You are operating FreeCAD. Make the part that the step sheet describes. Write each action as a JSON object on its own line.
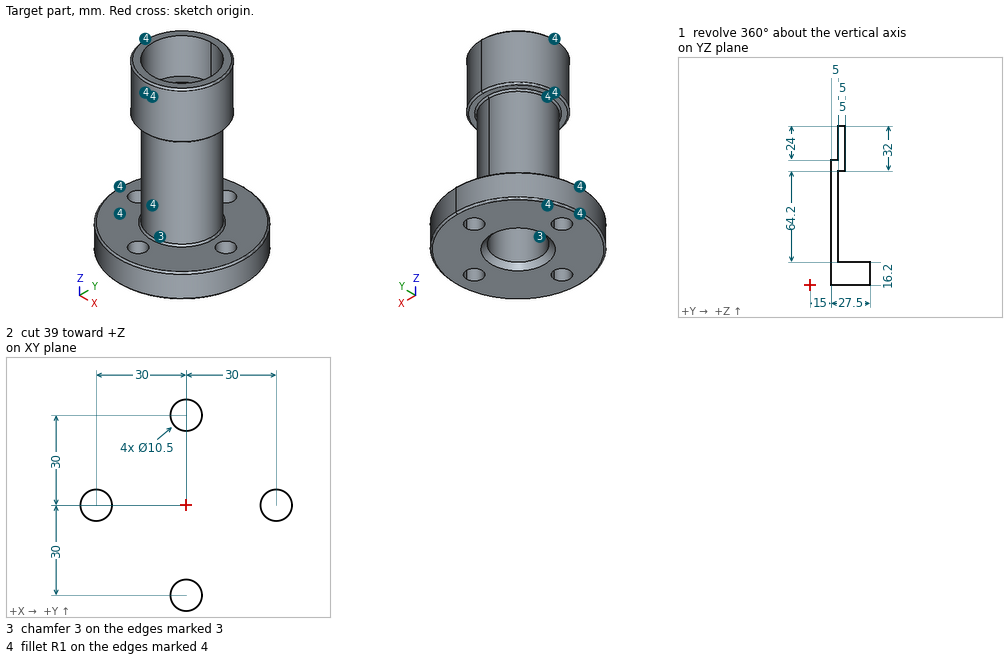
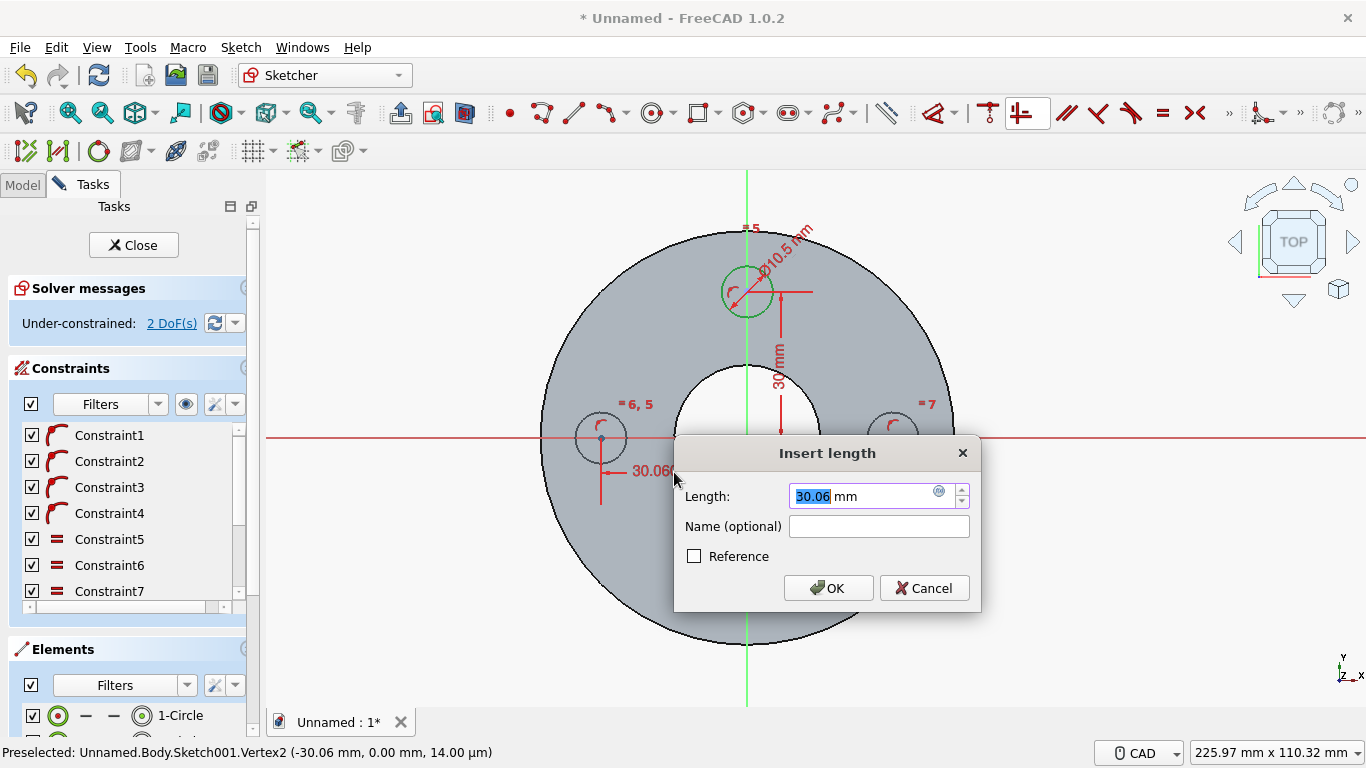
{"action": "type", "text": "30"}
{"action": "key", "text": "Return"}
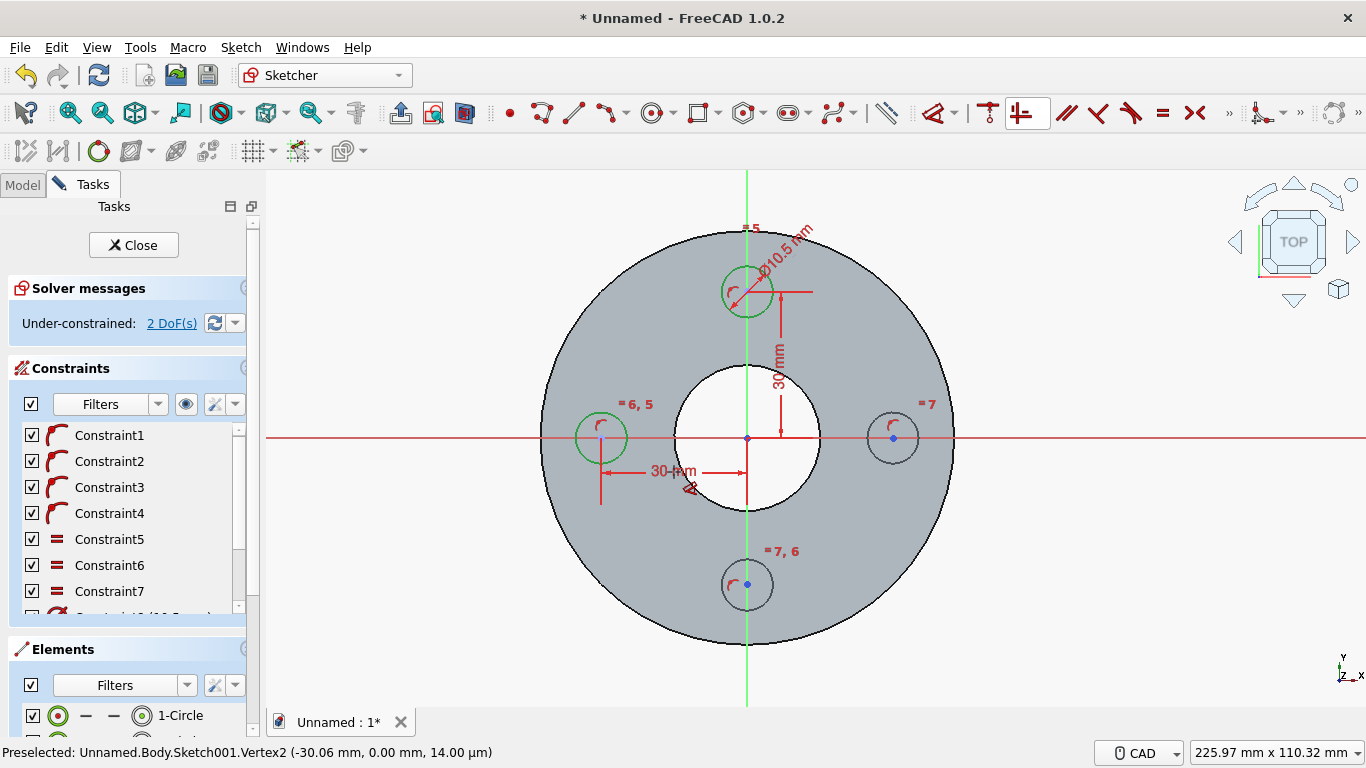
{"action": "left_click", "coordinate": [747, 585]}
{"action": "left_click", "coordinate": [781, 512]}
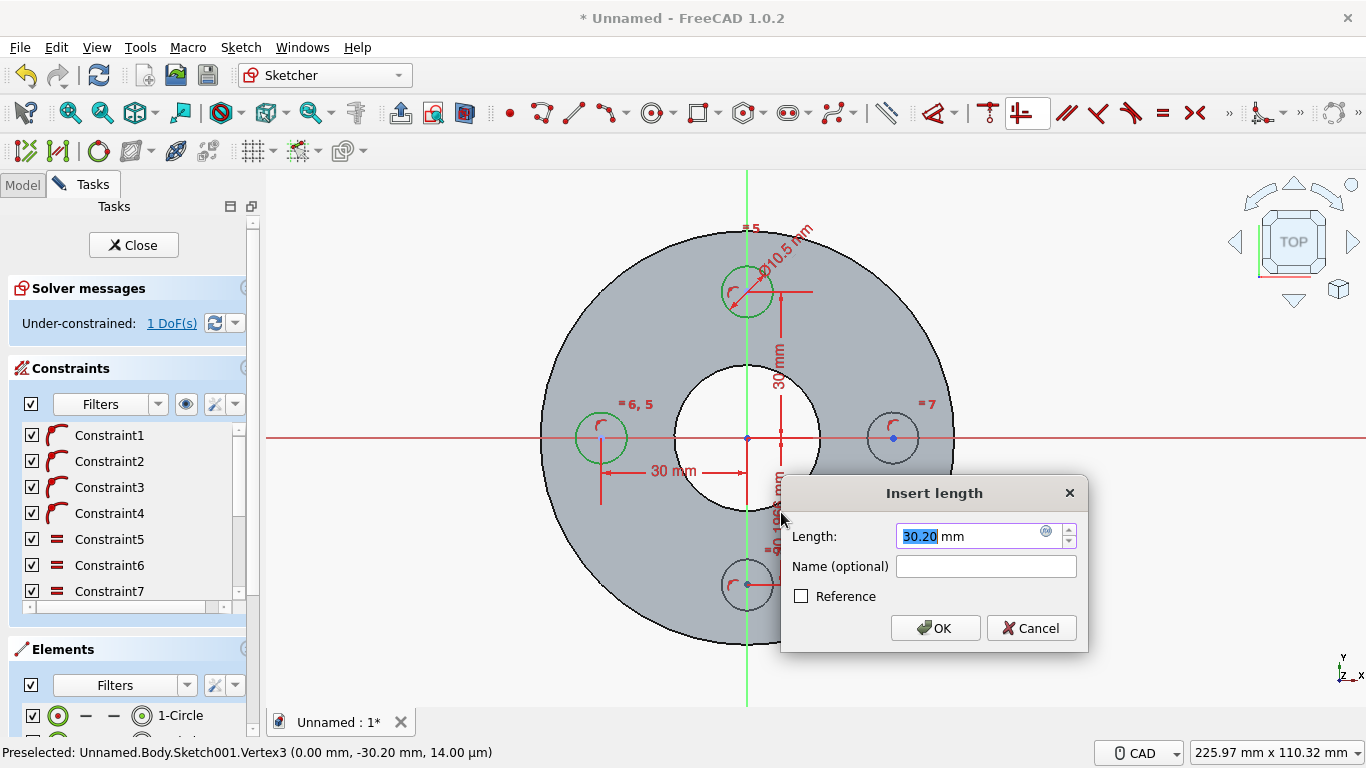
{"action": "type", "text": "30"}
{"action": "key", "text": "Return"}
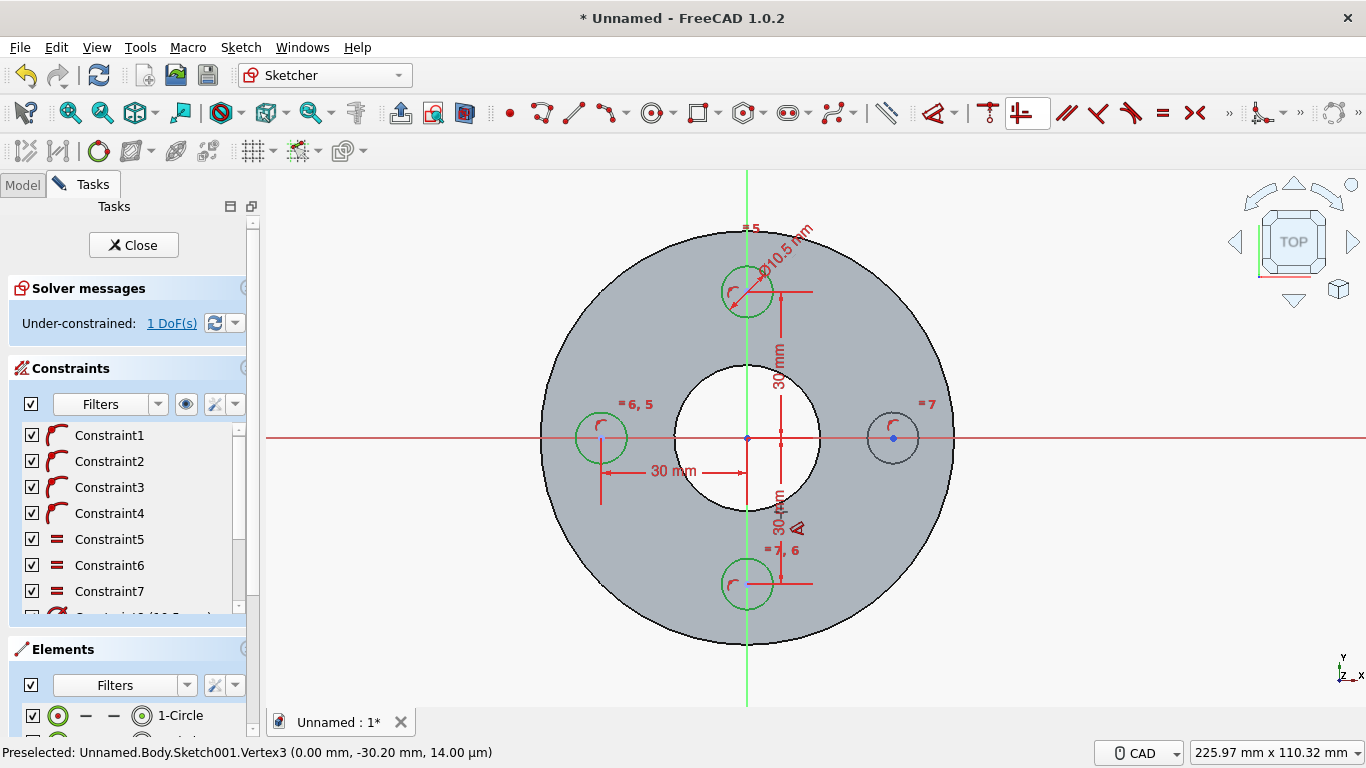
{"action": "left_click", "coordinate": [893, 438]}
{"action": "left_click", "coordinate": [820, 472]}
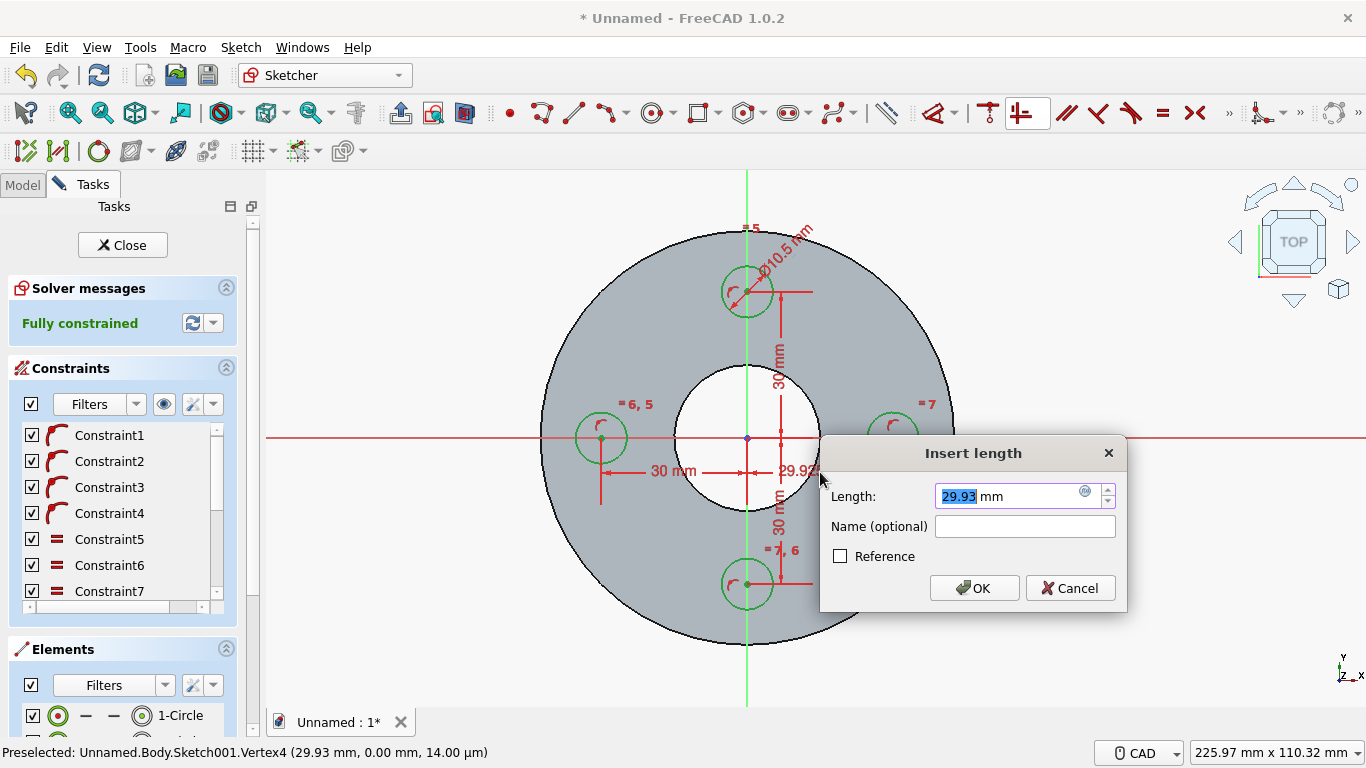
{"action": "type", "text": "30"}
{"action": "key", "text": "Return"}
{"action": "key", "text": "Escape"}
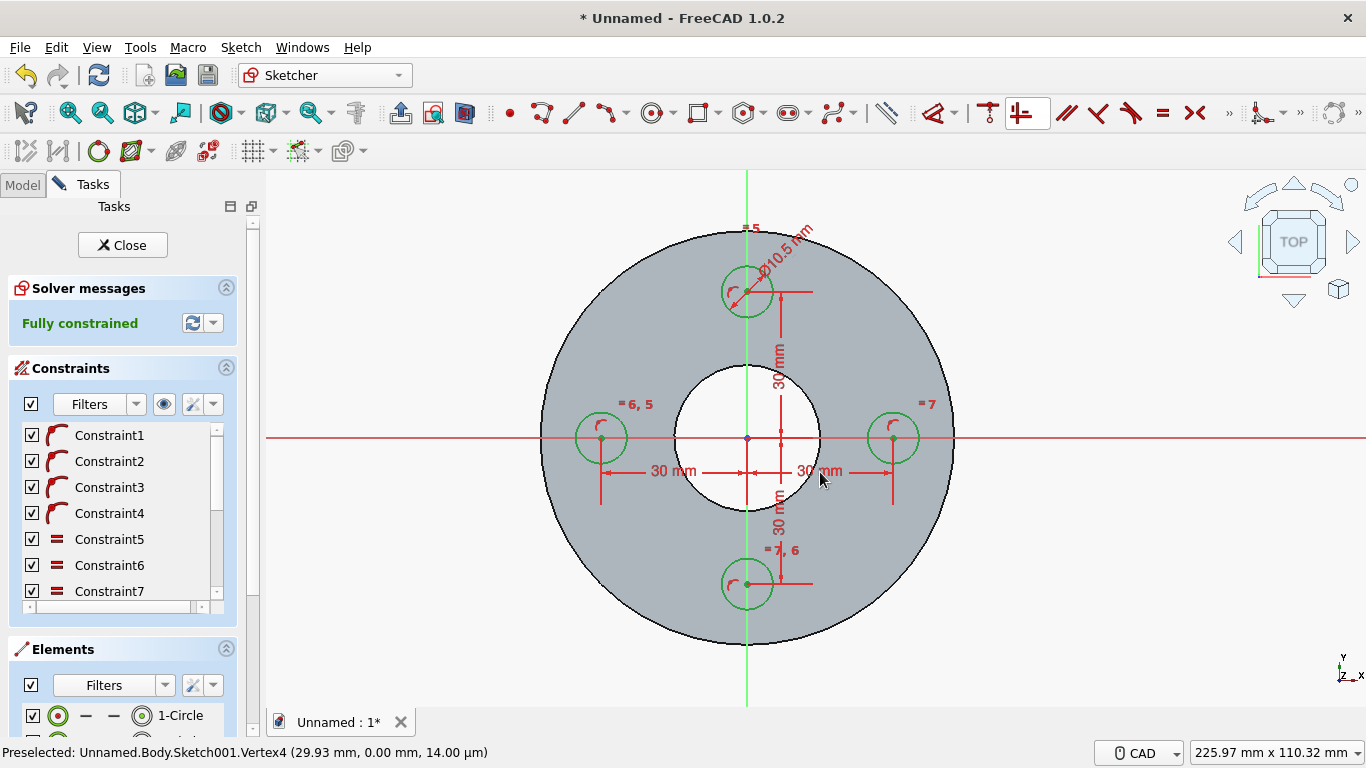
{"action": "left_click", "coordinate": [123, 245]}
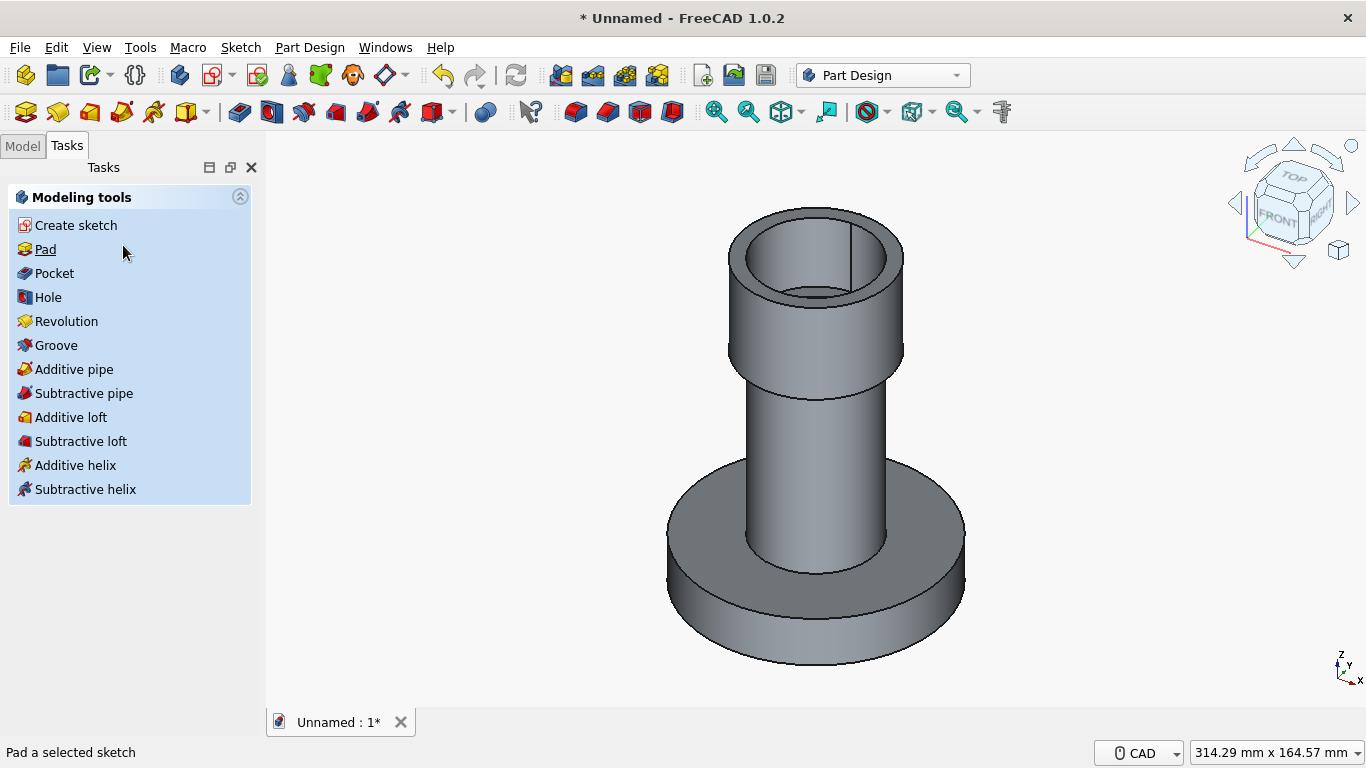
{"action": "left_click", "coordinate": [240, 112]}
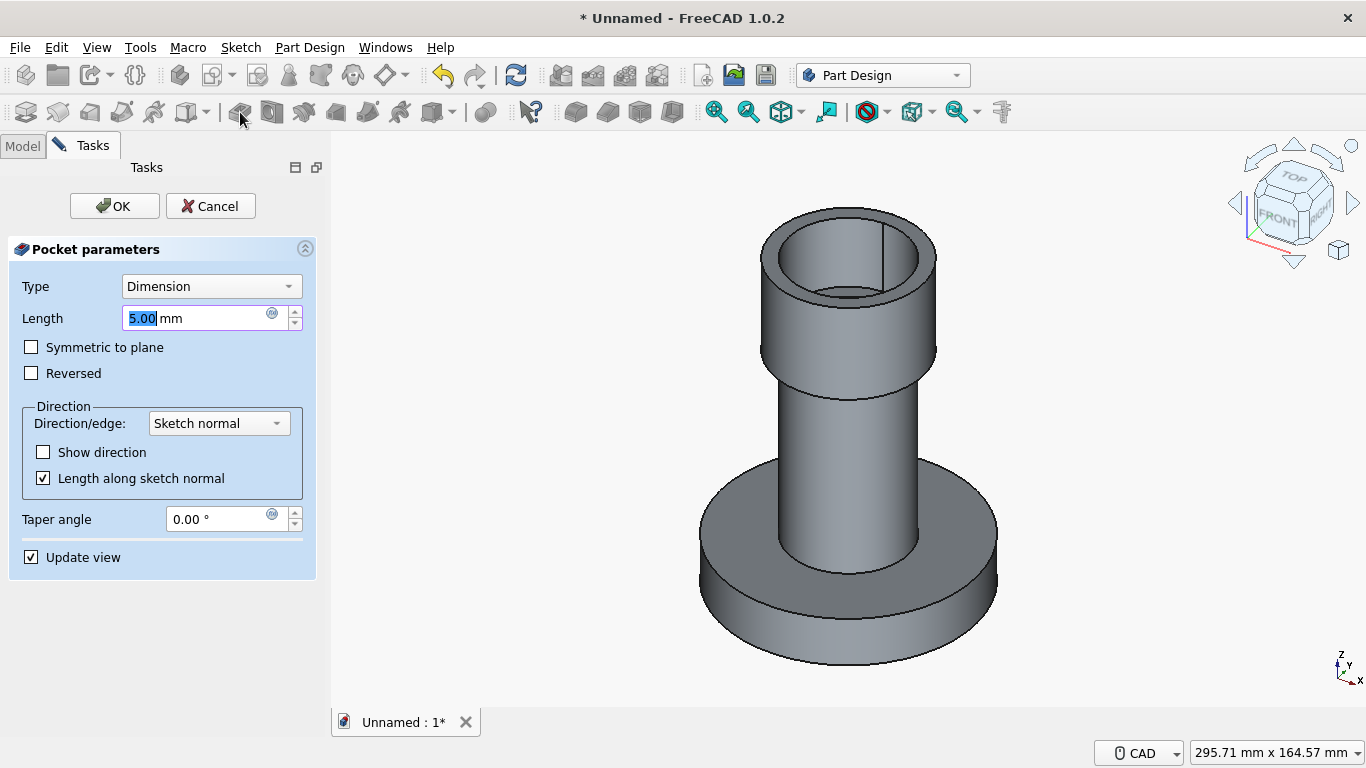
{"action": "type", "text": "39"}
{"action": "key", "text": "Tab"}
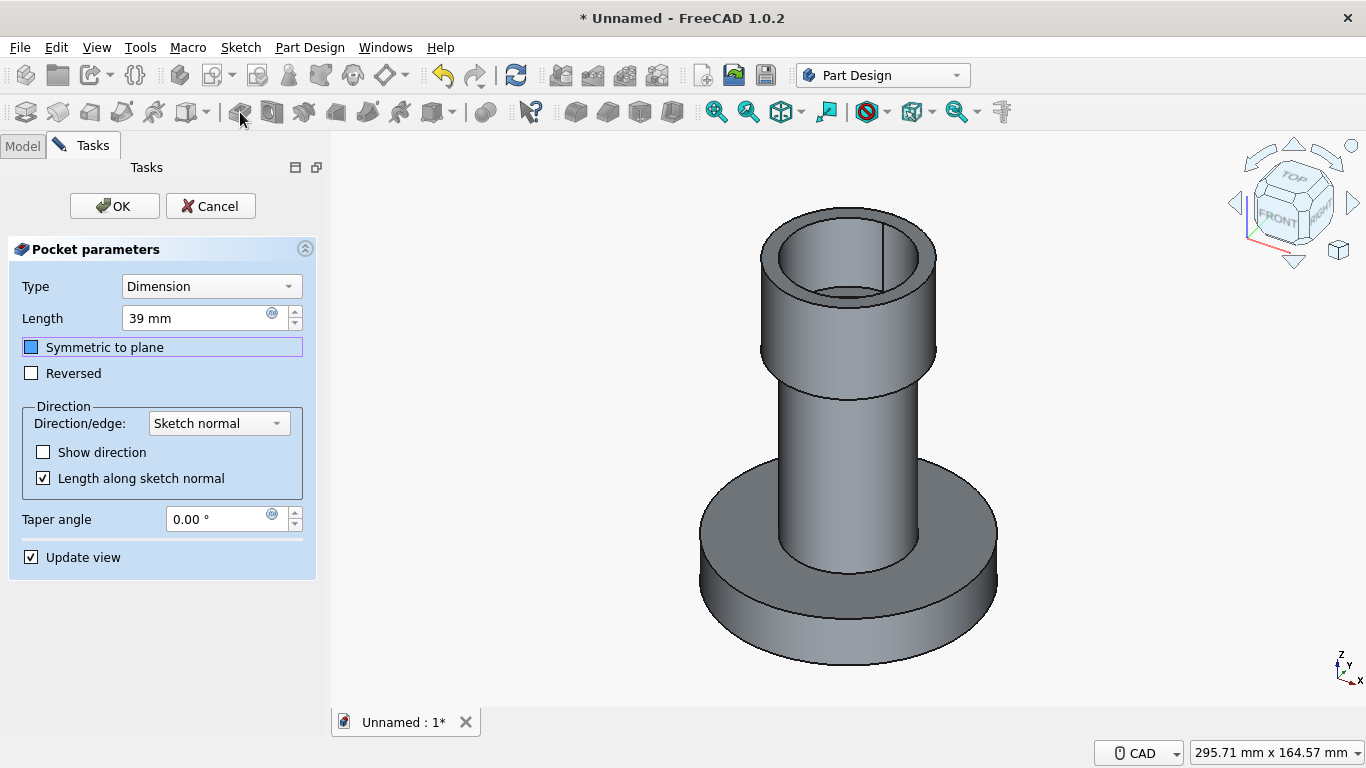
{"action": "left_click", "coordinate": [30, 373]}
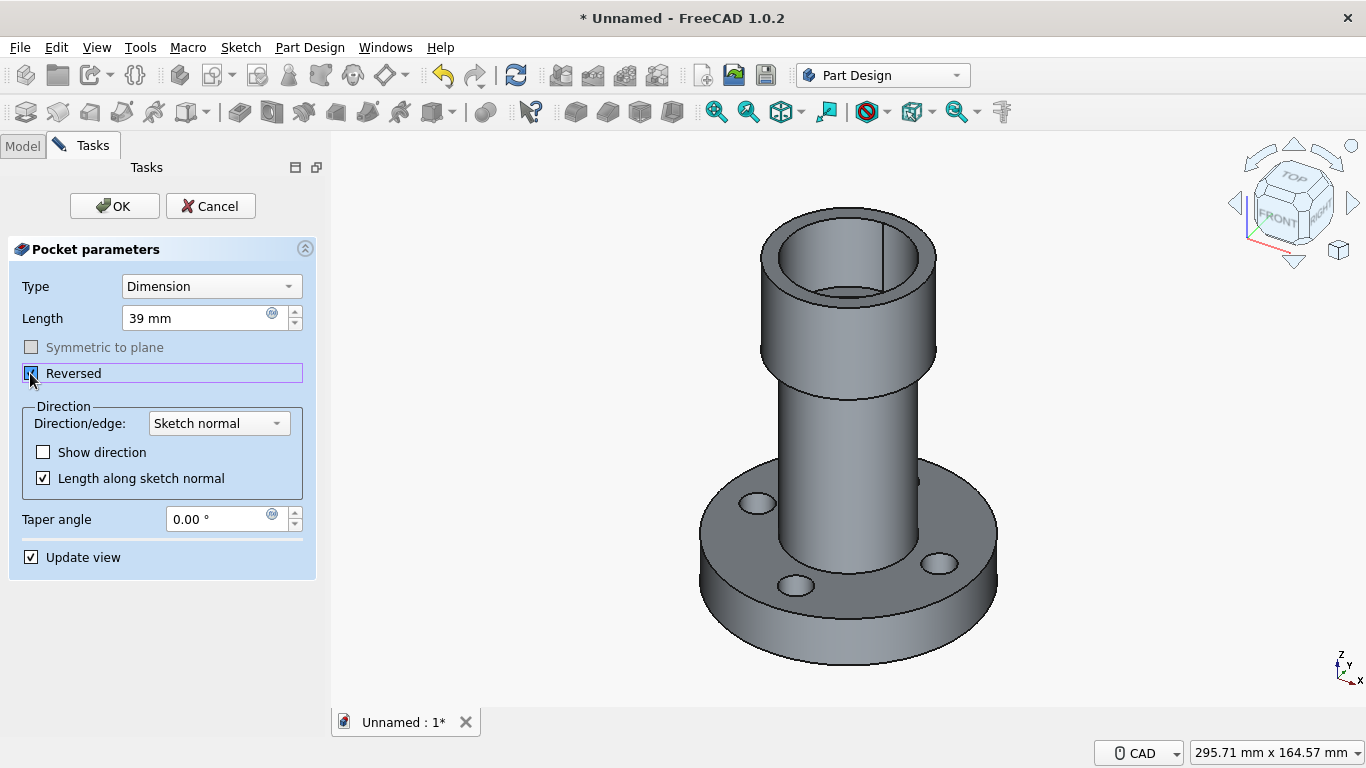
{"action": "left_click", "coordinate": [115, 206]}